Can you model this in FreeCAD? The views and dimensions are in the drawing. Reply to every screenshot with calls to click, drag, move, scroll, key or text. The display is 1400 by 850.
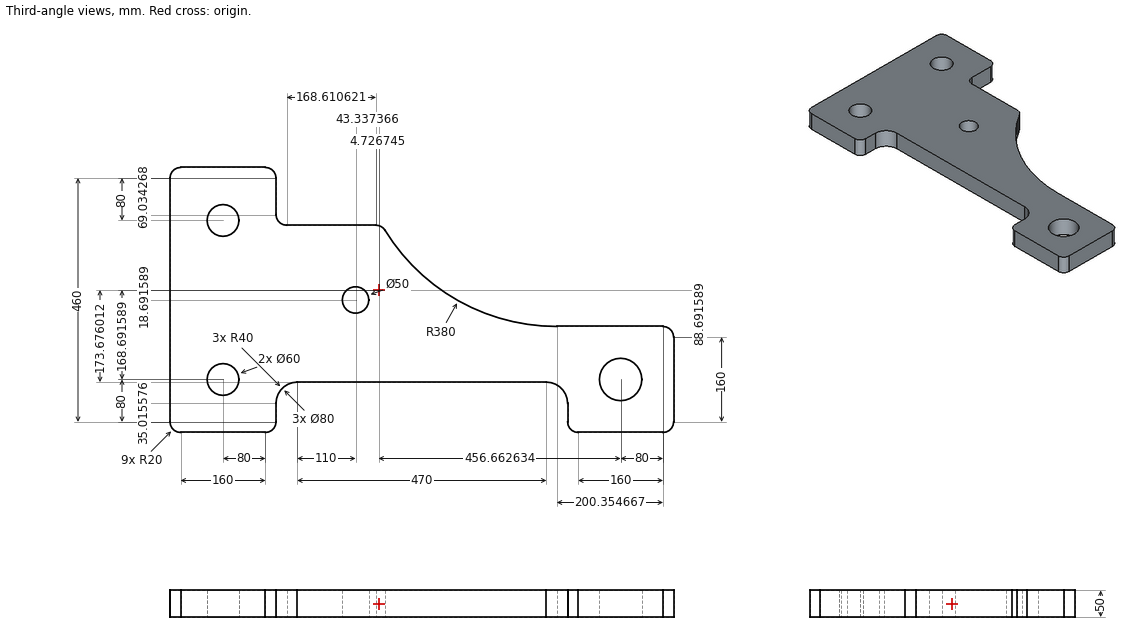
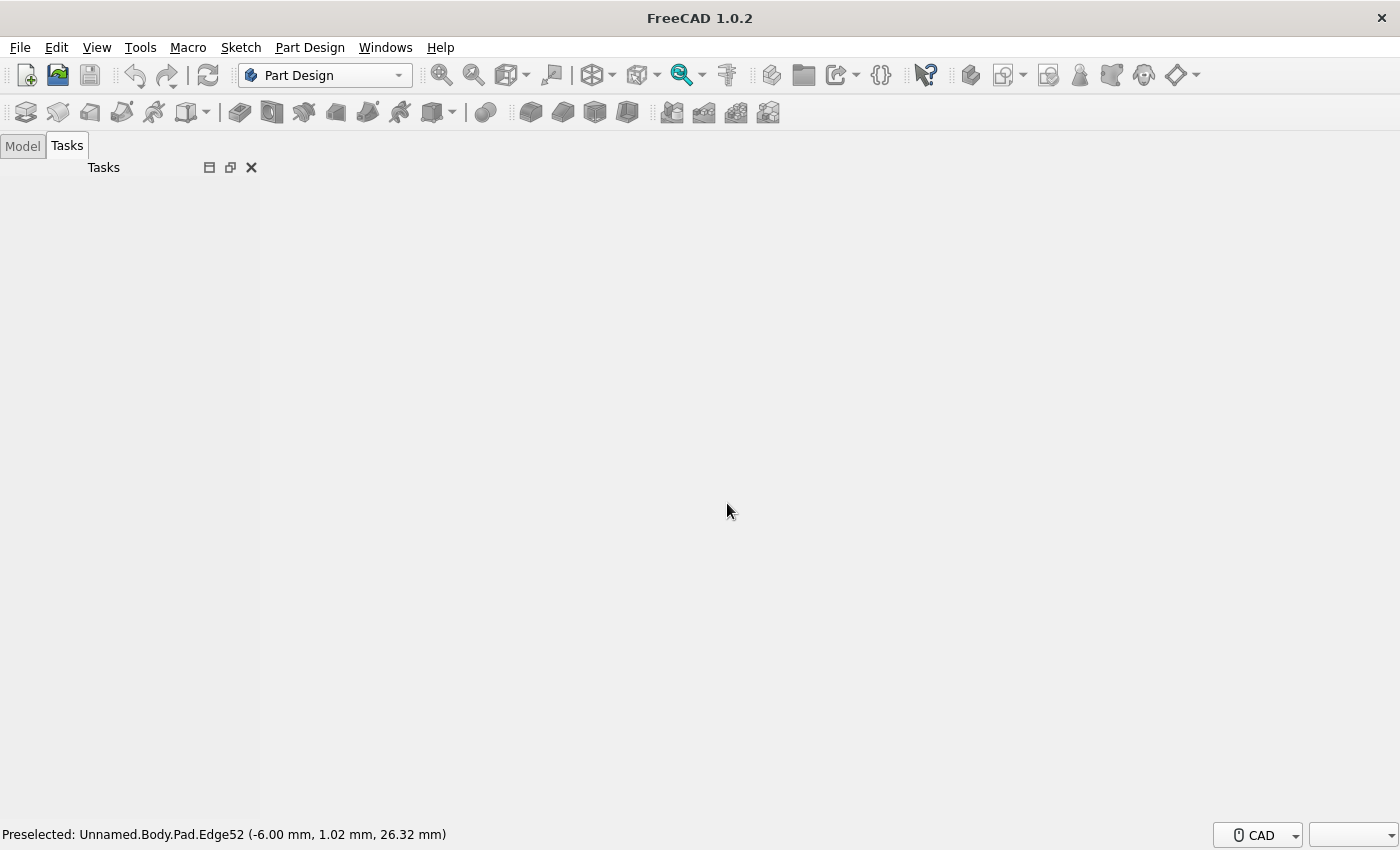
click(26, 76)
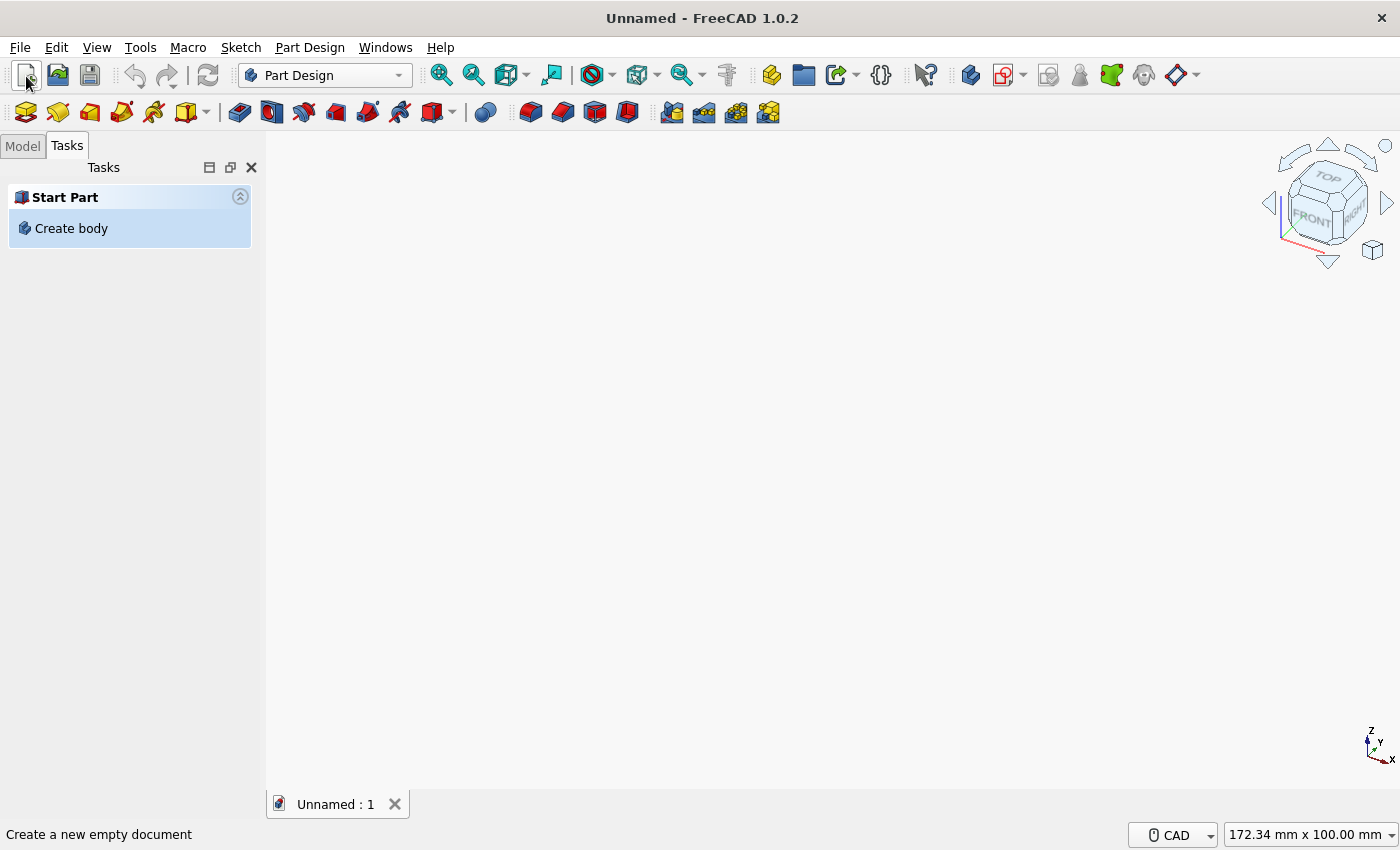
click(1004, 76)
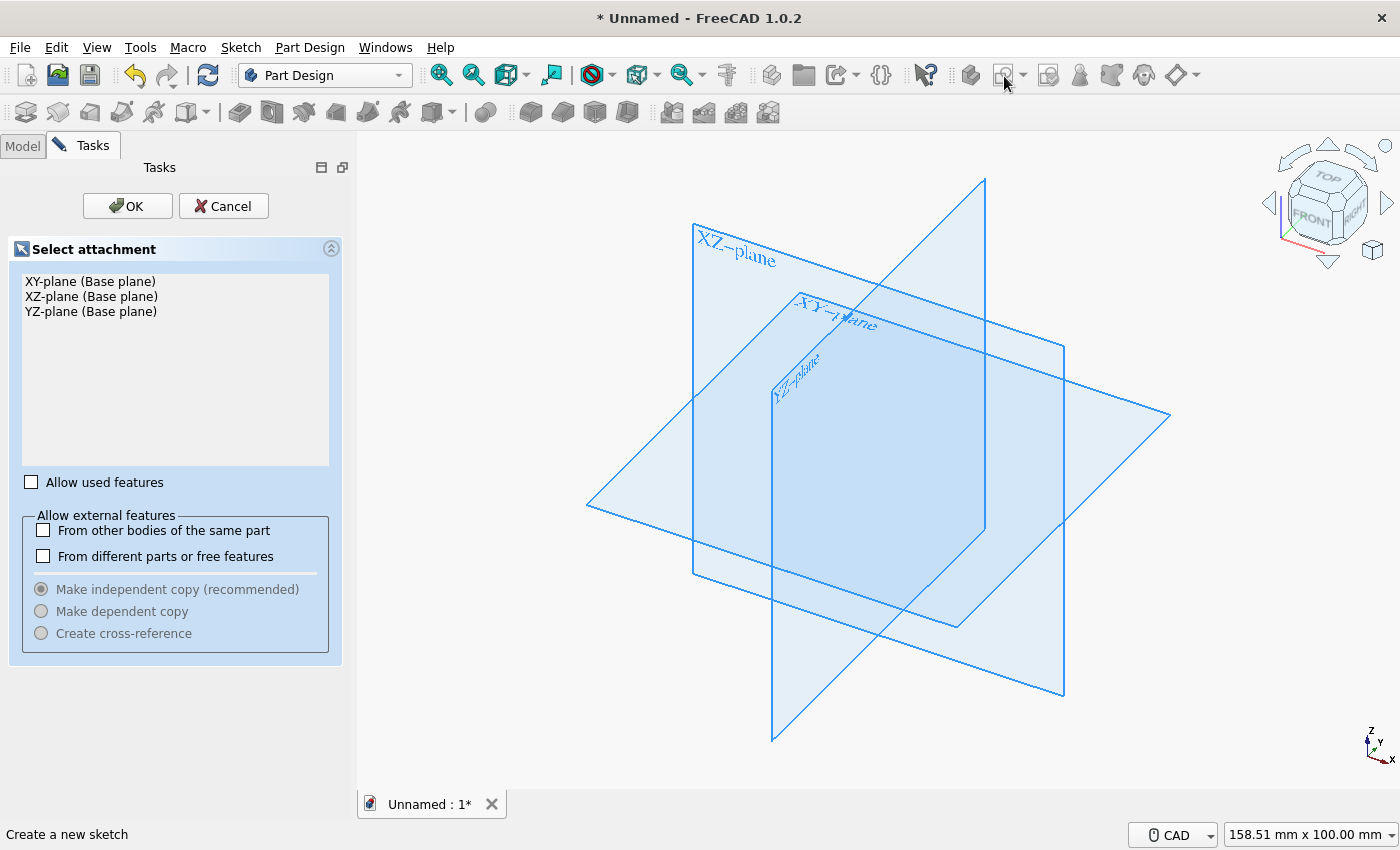
click(82, 282)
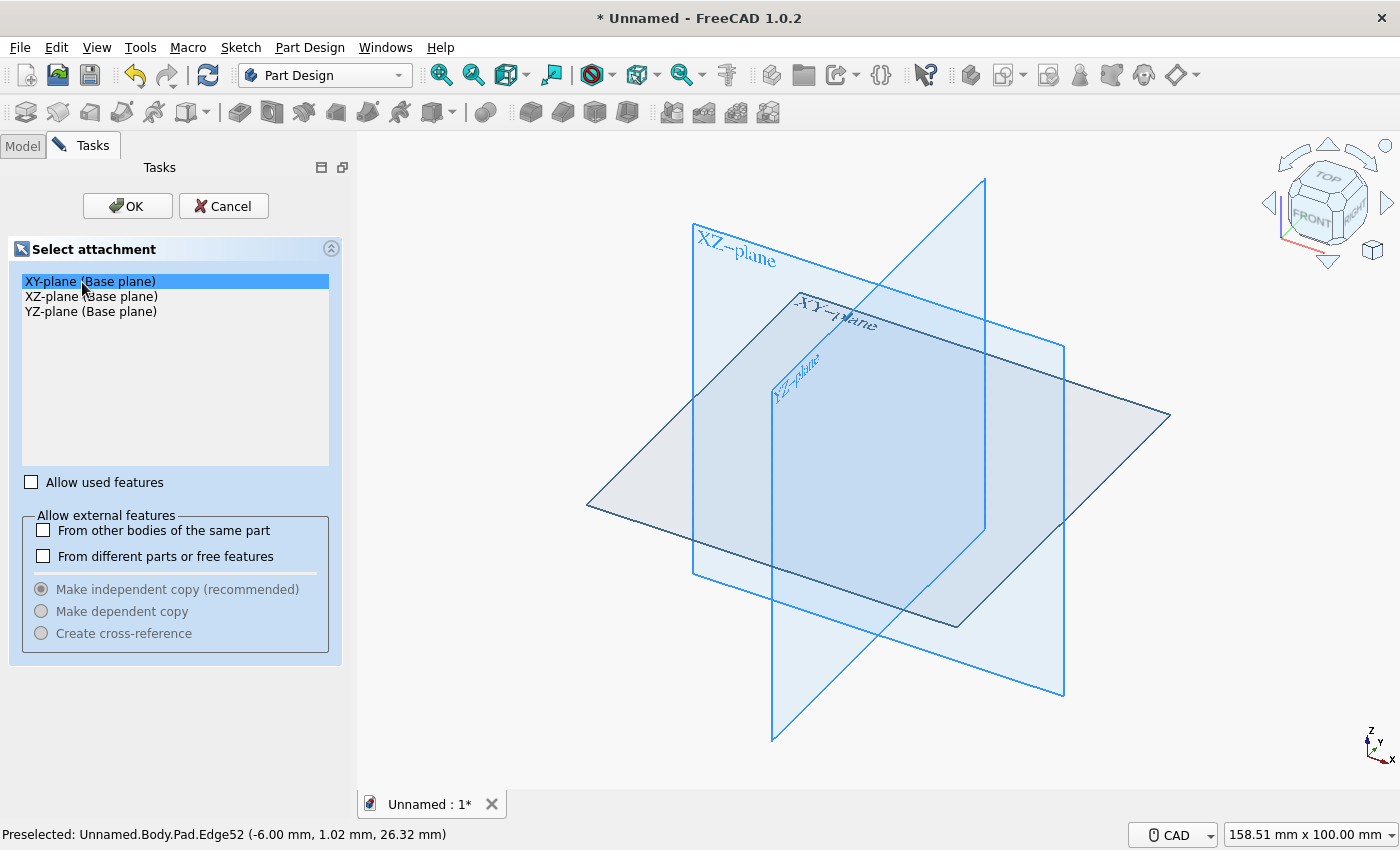
click(128, 206)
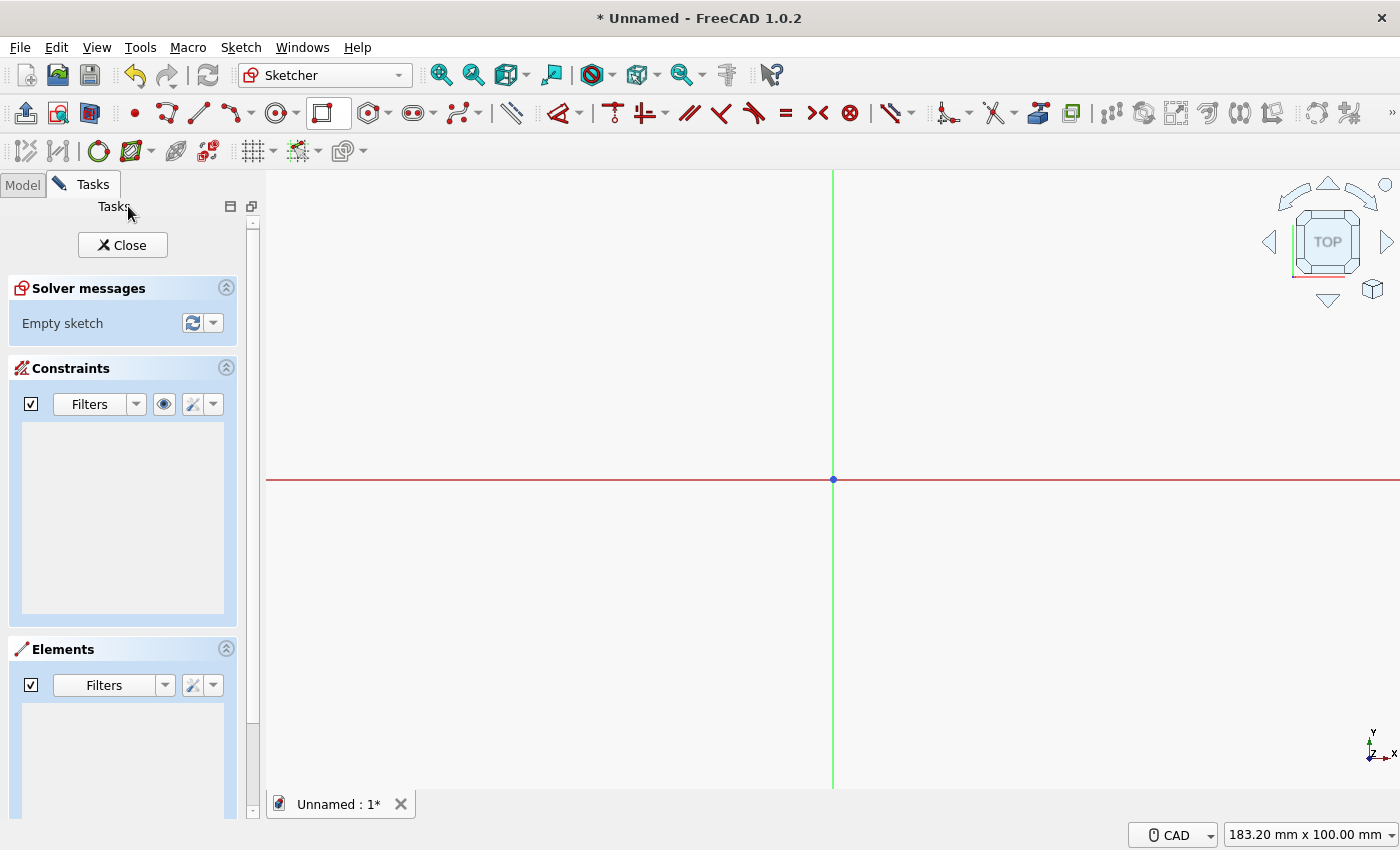
scroll(693, 465, down, 11)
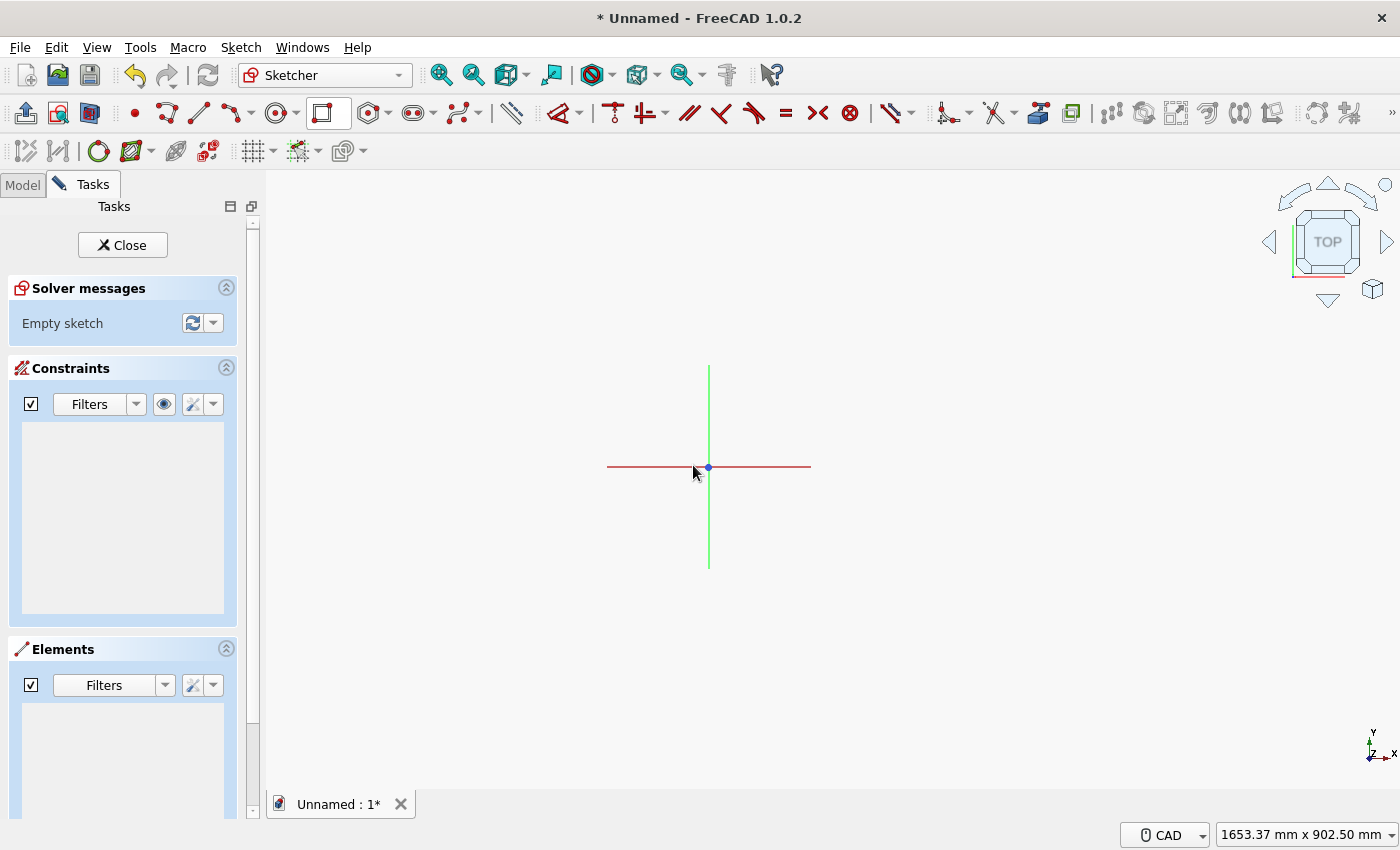
click(200, 114)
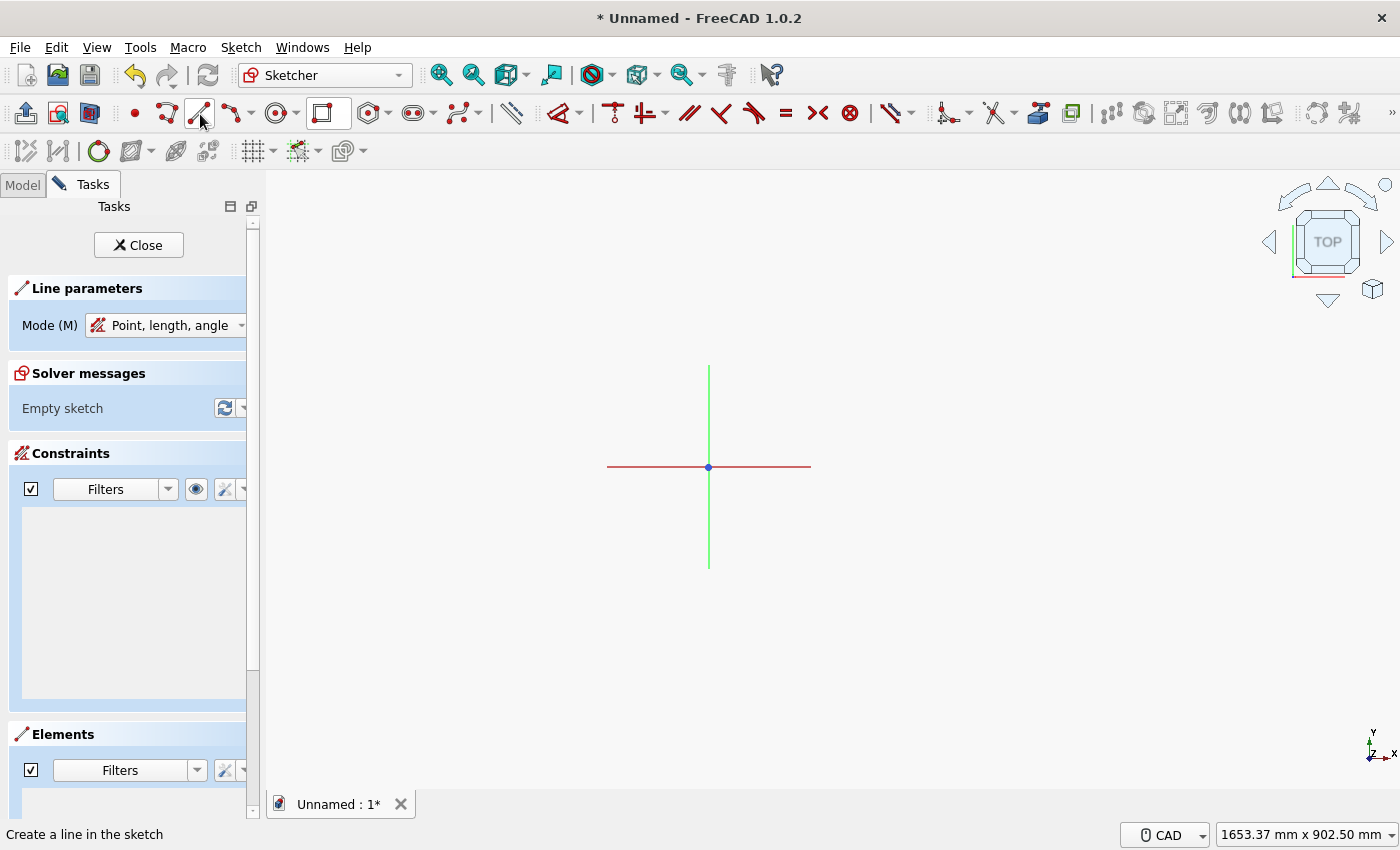
click(439, 322)
click(439, 638)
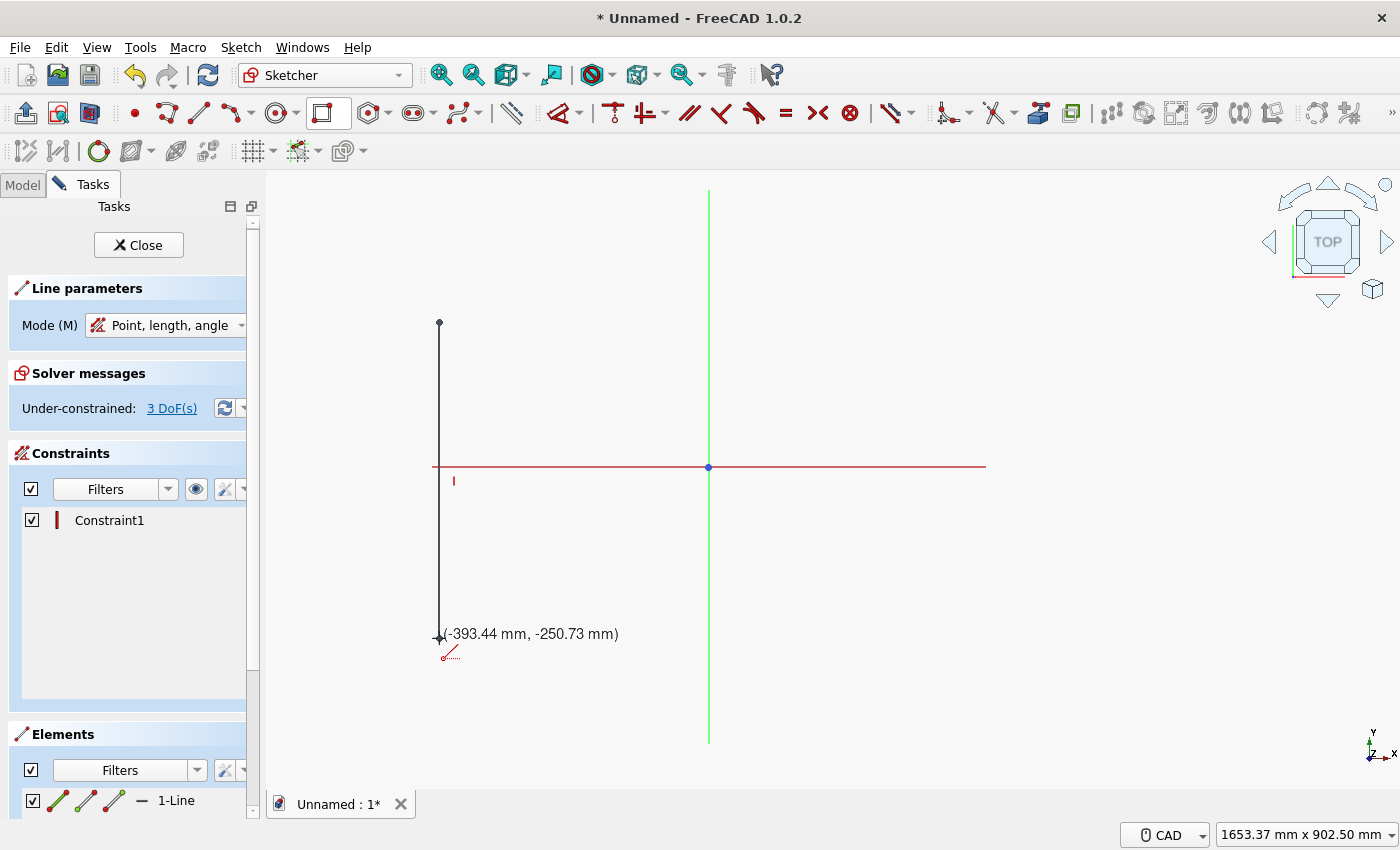
click(453, 651)
click(563, 651)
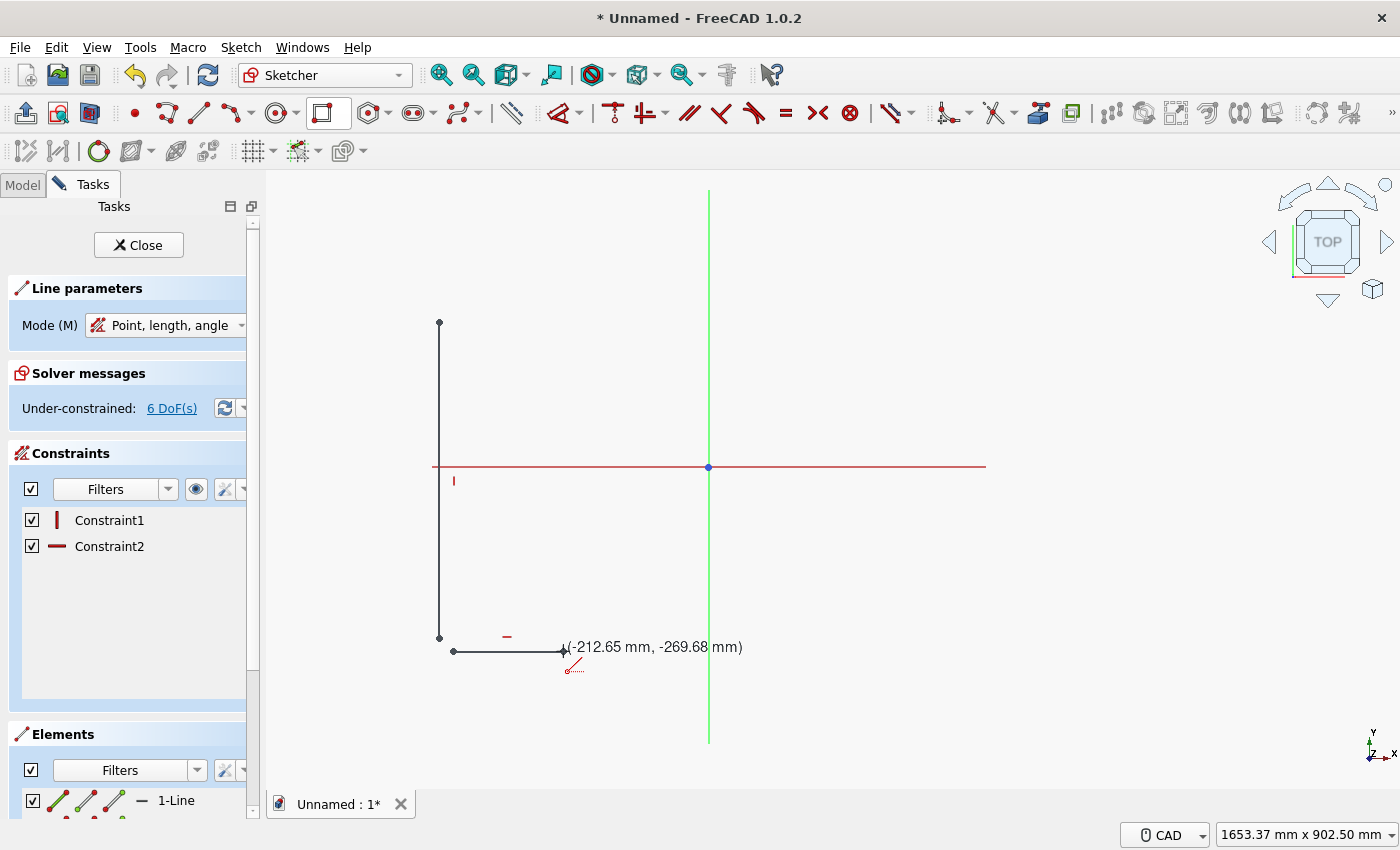
click(576, 638)
click(576, 614)